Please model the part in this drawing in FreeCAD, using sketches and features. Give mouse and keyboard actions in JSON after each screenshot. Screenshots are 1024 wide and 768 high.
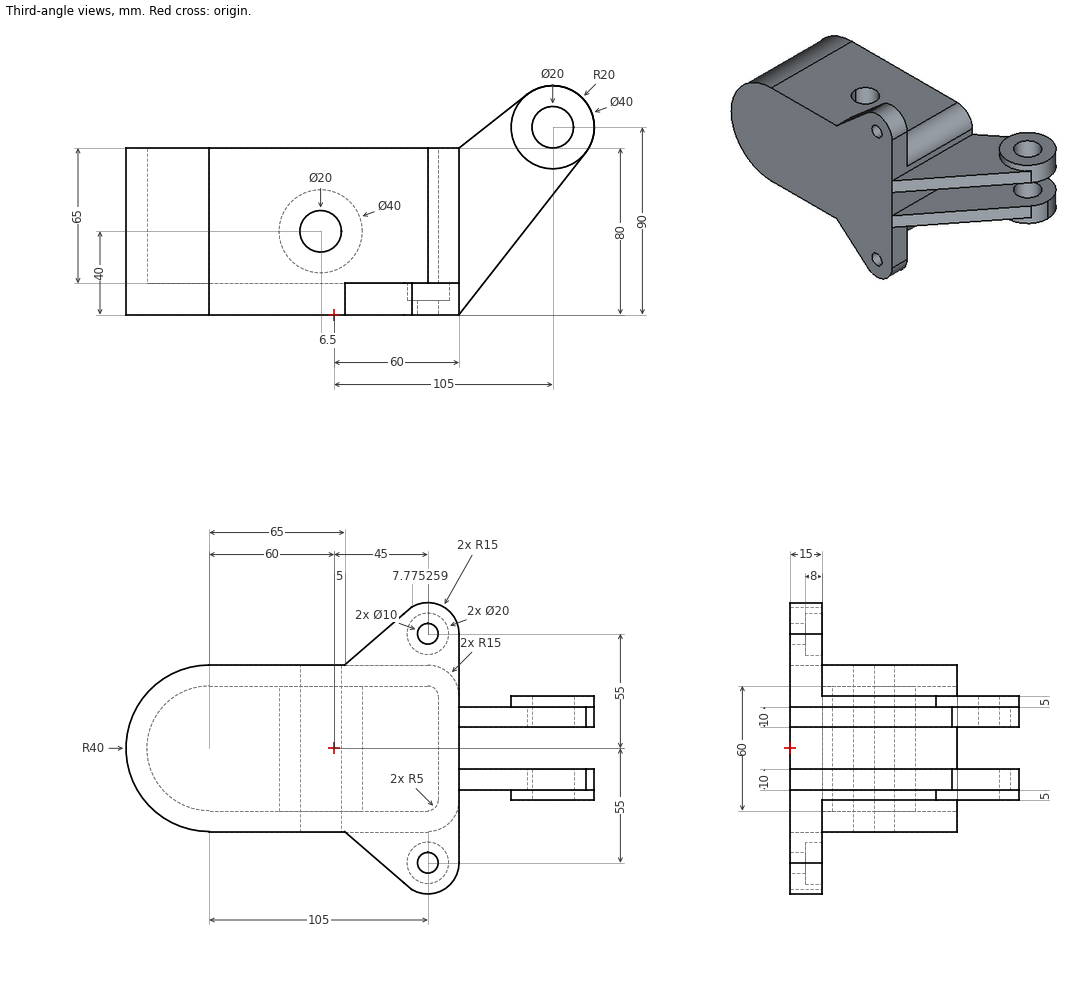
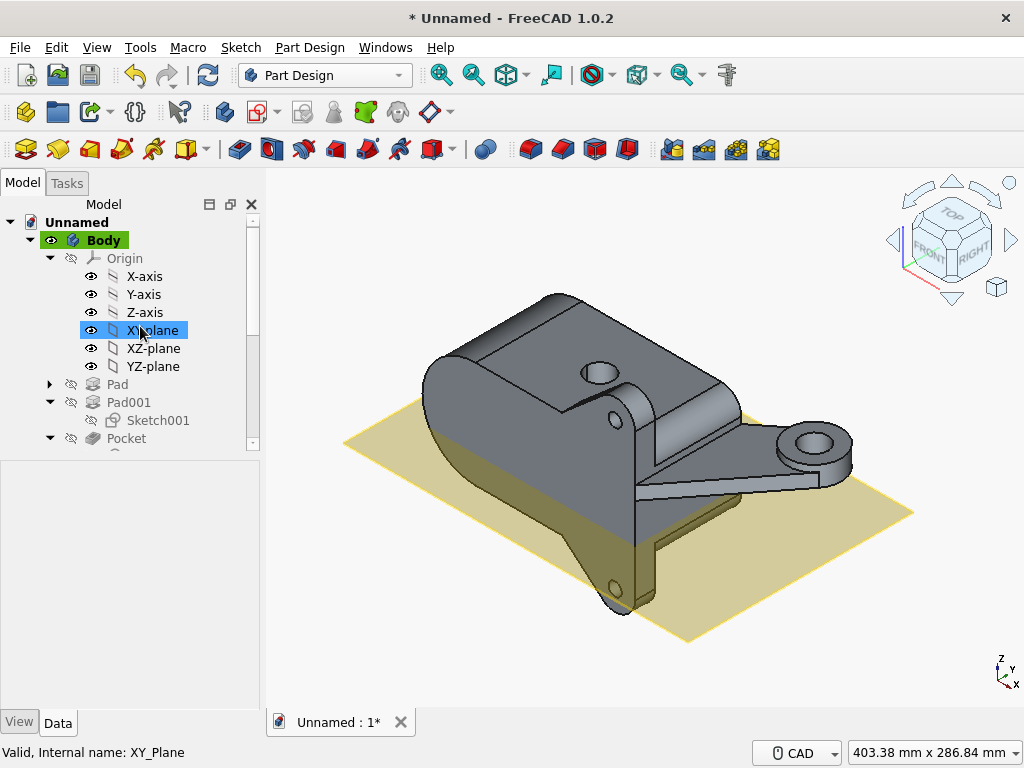
{"action": "scroll", "coordinate": [100, 326], "scroll_direction": "down", "scroll_amount": 6}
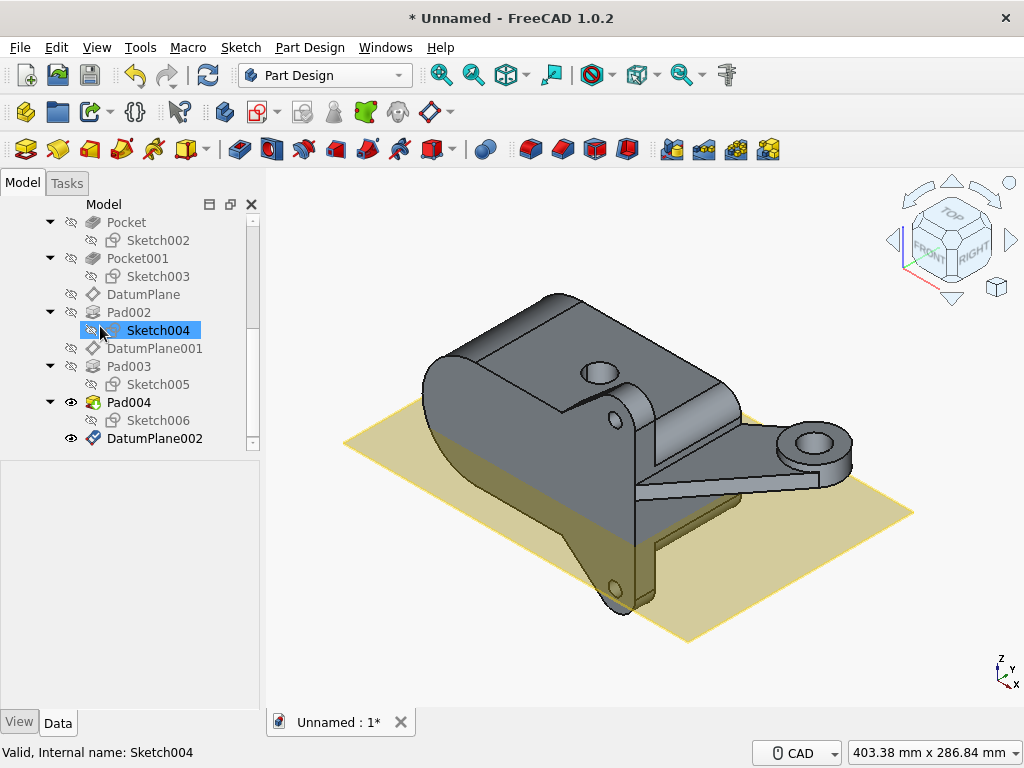
{"action": "left_click", "coordinate": [116, 438]}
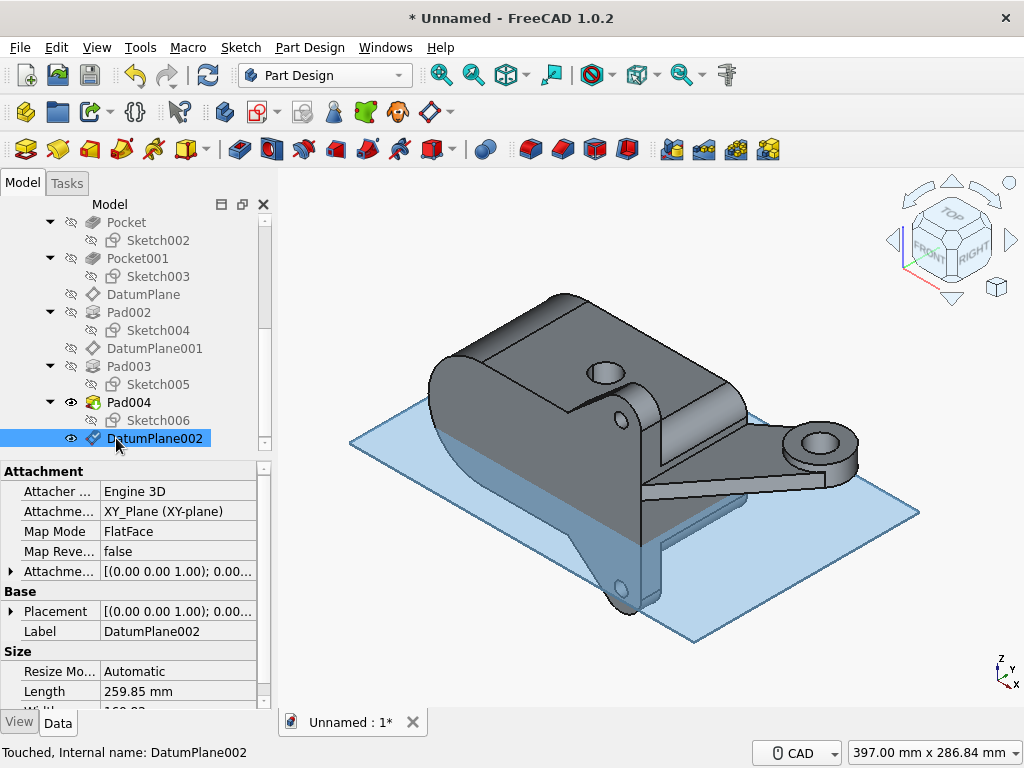
{"action": "left_click", "coordinate": [258, 112]}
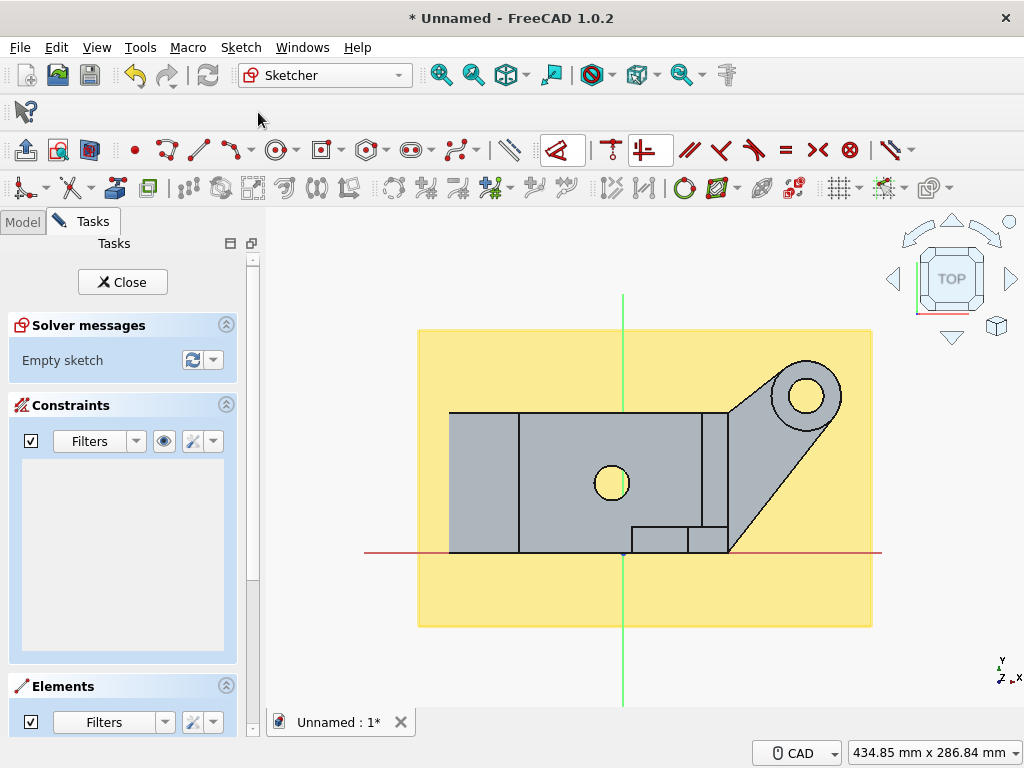
{"action": "left_click", "coordinate": [90, 150]}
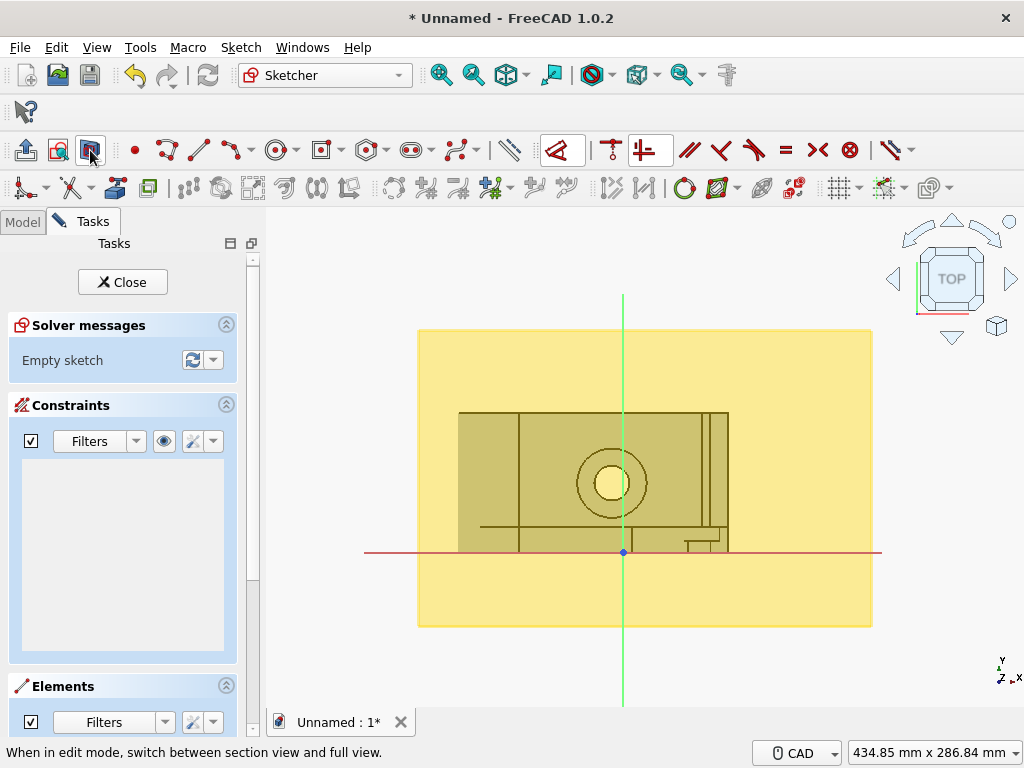
{"action": "scroll", "coordinate": [859, 465], "scroll_direction": "up", "scroll_amount": 3}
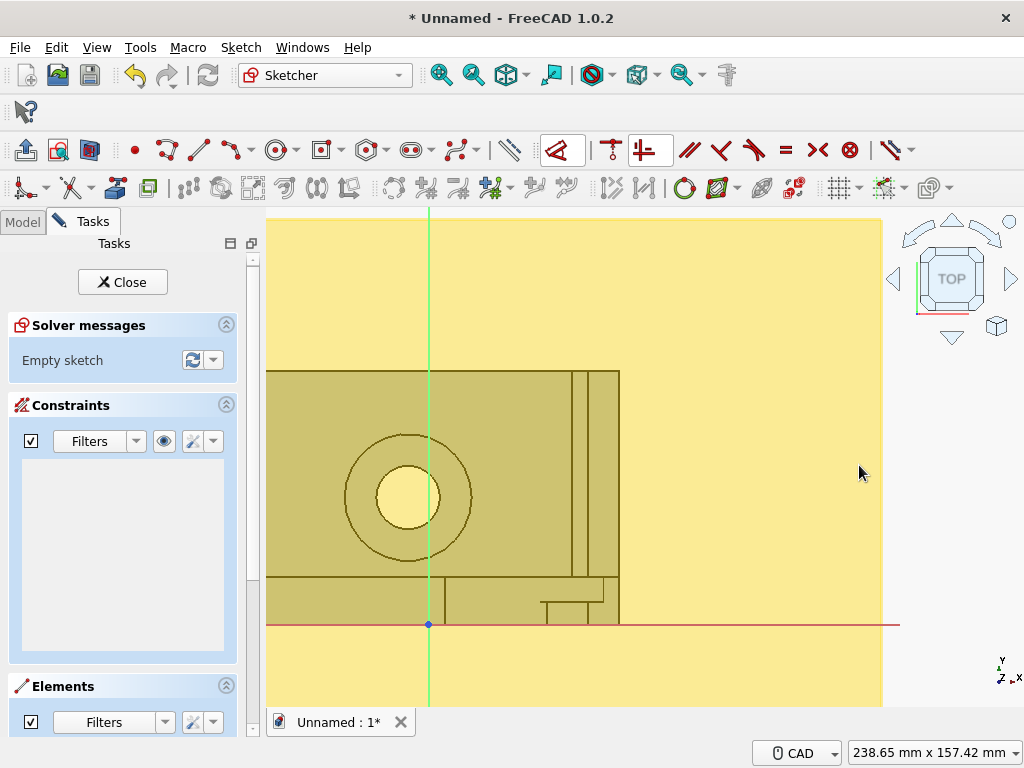
{"action": "left_click", "coordinate": [168, 150]}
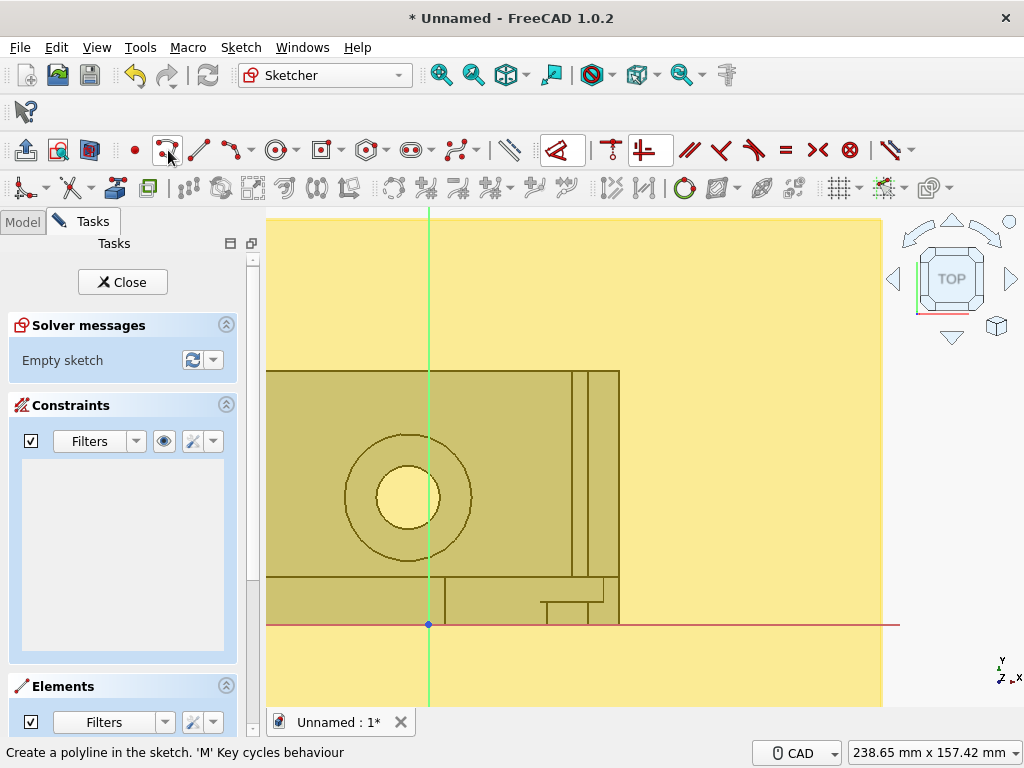
{"action": "left_click", "coordinate": [723, 289]}
{"action": "left_click", "coordinate": [619, 371]}
{"action": "left_click", "coordinate": [619, 625]}
{"action": "left_click", "coordinate": [812, 378]}
{"action": "right_click", "coordinate": [812, 378]}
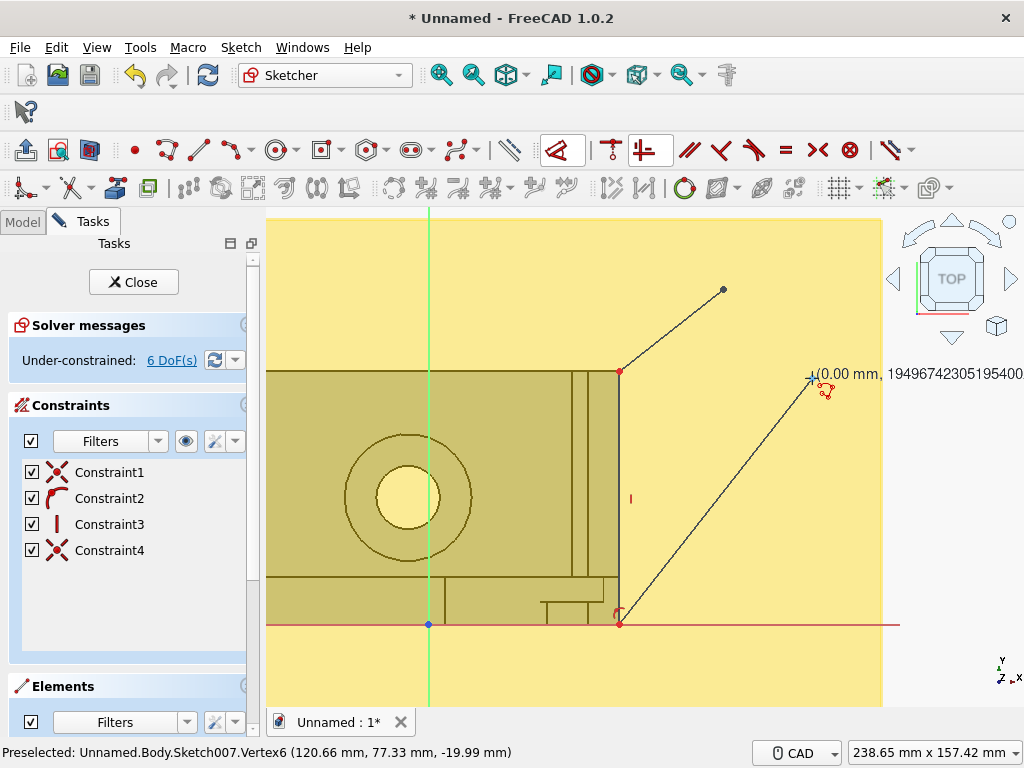
{"action": "left_click", "coordinate": [232, 150]}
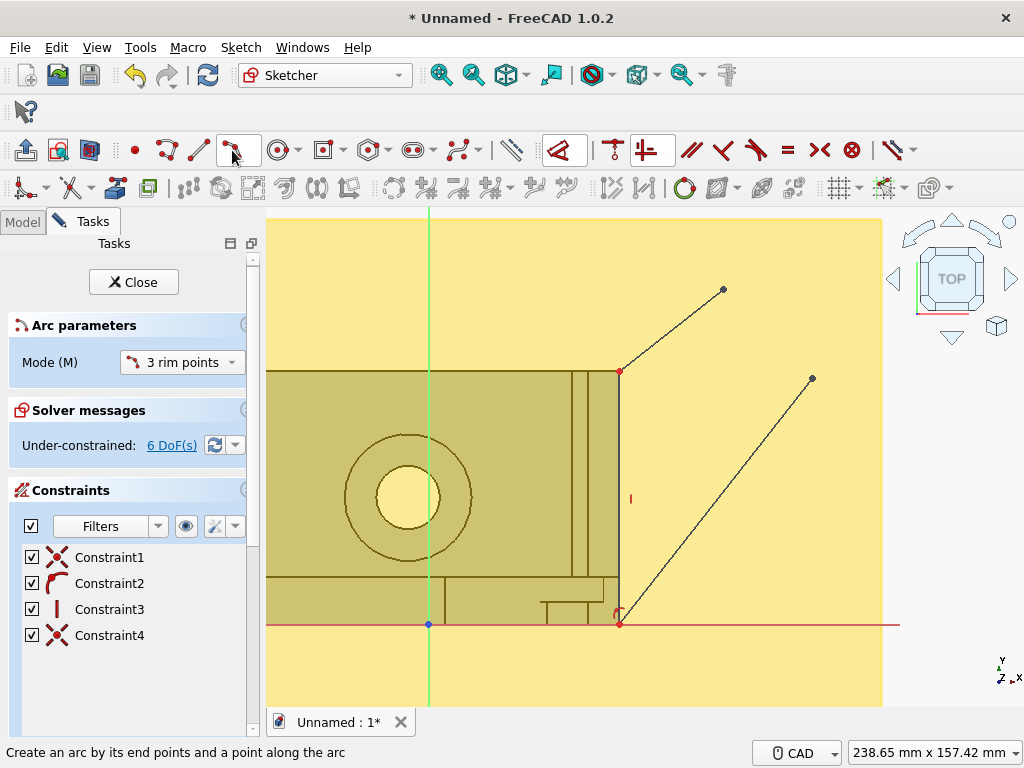
{"action": "left_click", "coordinate": [812, 379]}
{"action": "left_click", "coordinate": [723, 290]}
{"action": "left_click", "coordinate": [807, 294]}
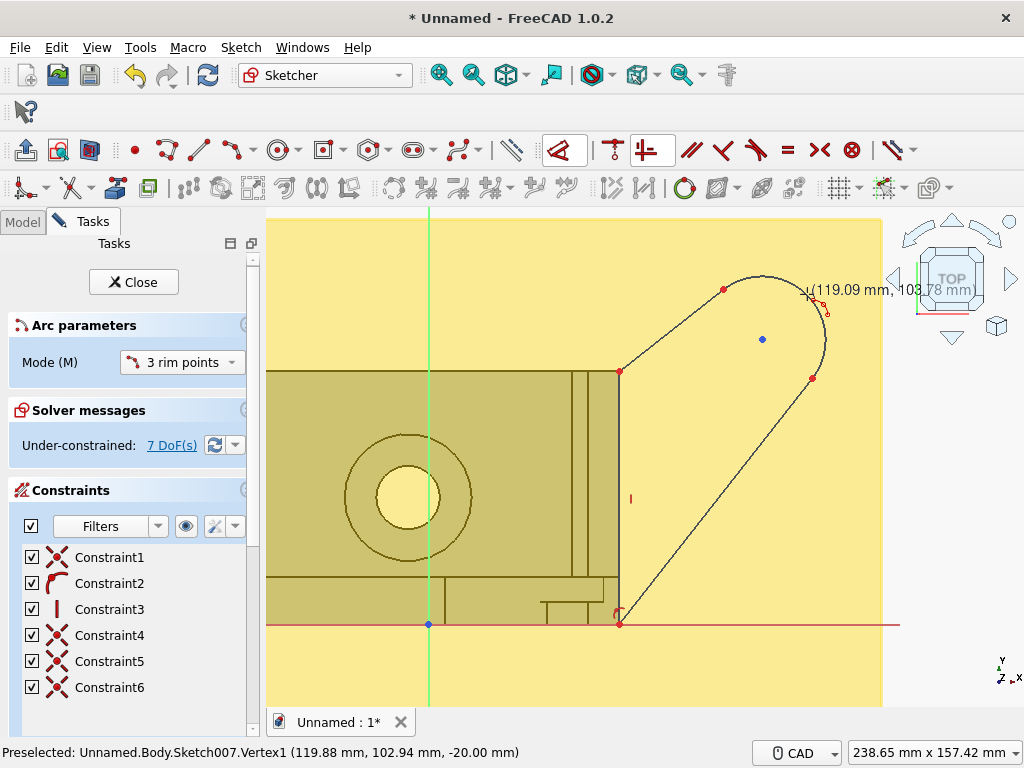
{"action": "left_click", "coordinate": [278, 150]}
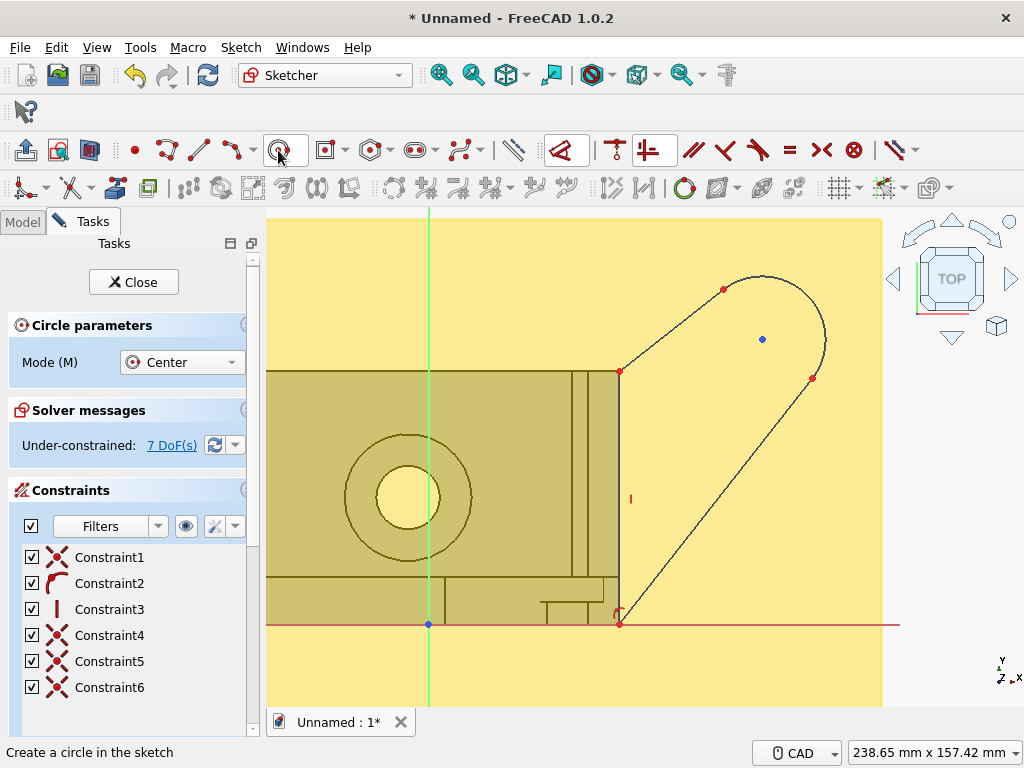
{"action": "left_click", "coordinate": [762, 339]}
{"action": "left_click", "coordinate": [785, 316]}
{"action": "key", "text": "Escape"}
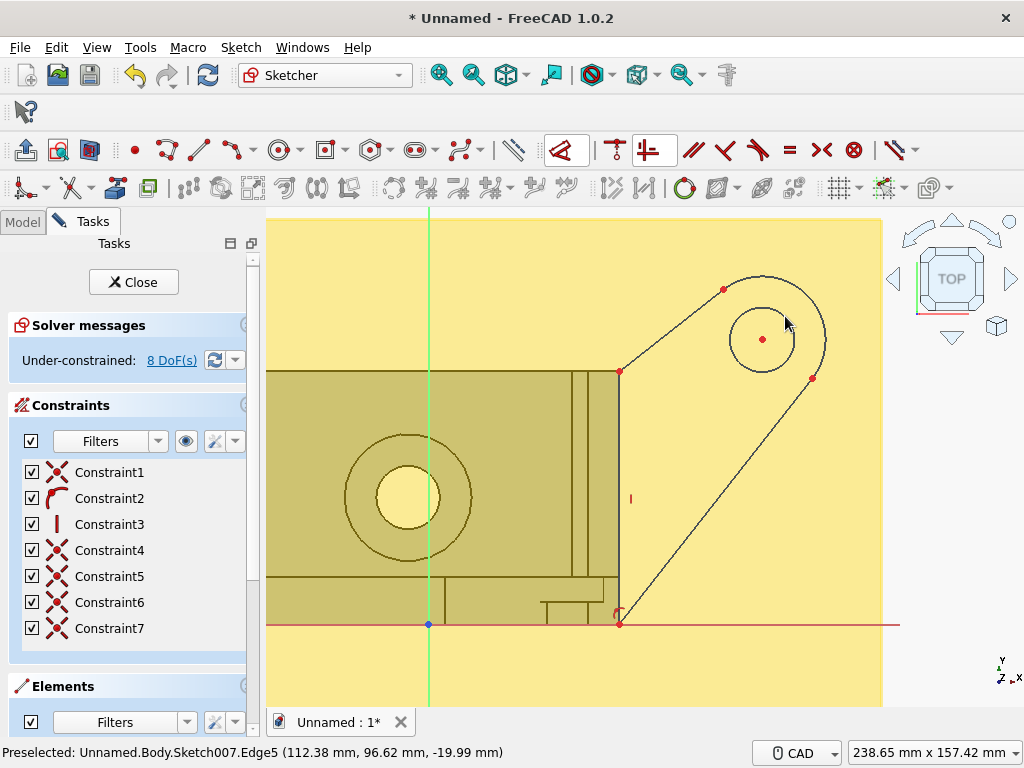
{"action": "left_click", "coordinate": [692, 315]}